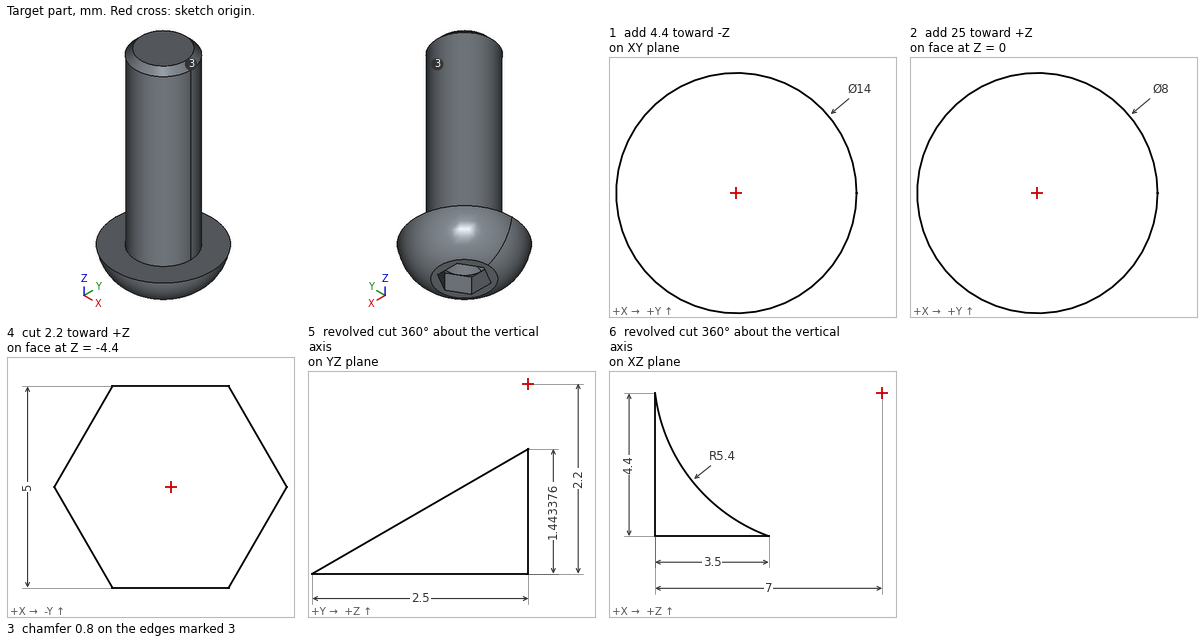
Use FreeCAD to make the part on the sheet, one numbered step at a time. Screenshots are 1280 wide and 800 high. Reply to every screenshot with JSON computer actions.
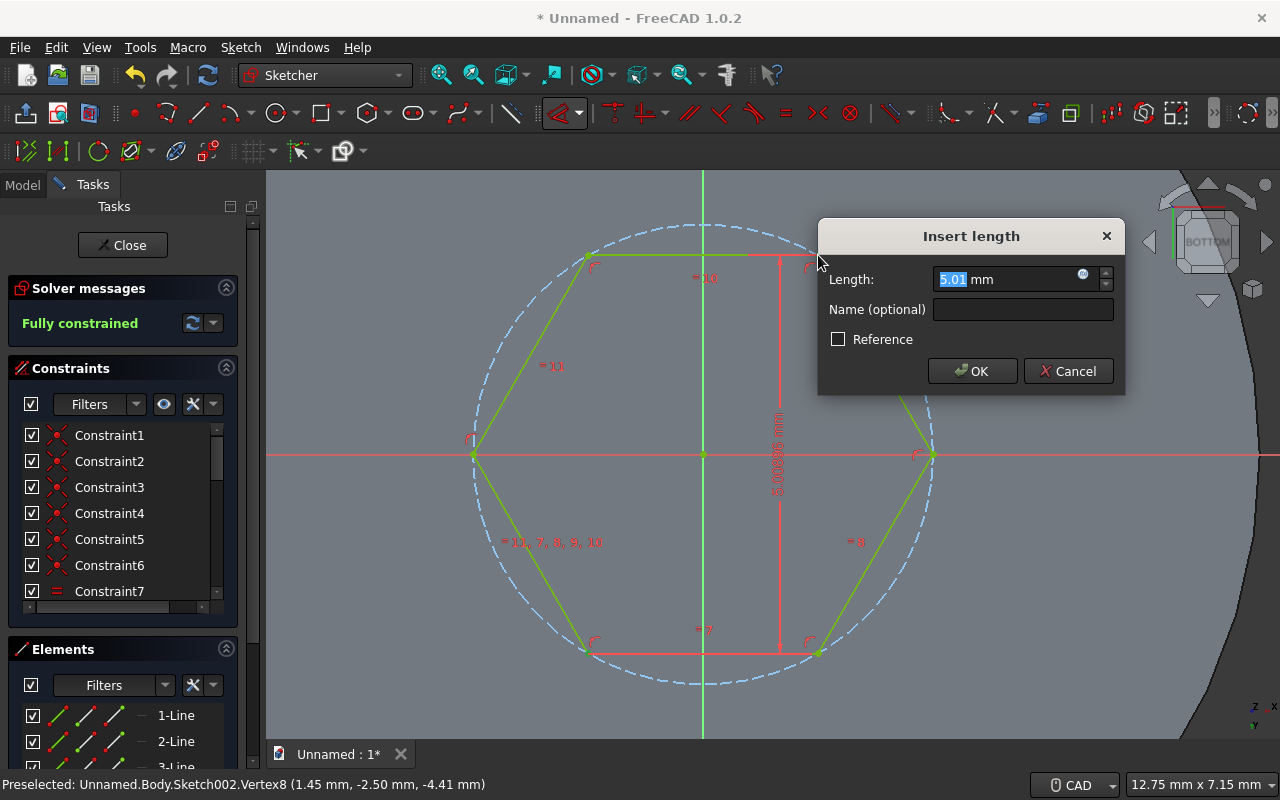
{"action": "type", "text": "5"}
{"action": "key", "text": "Return"}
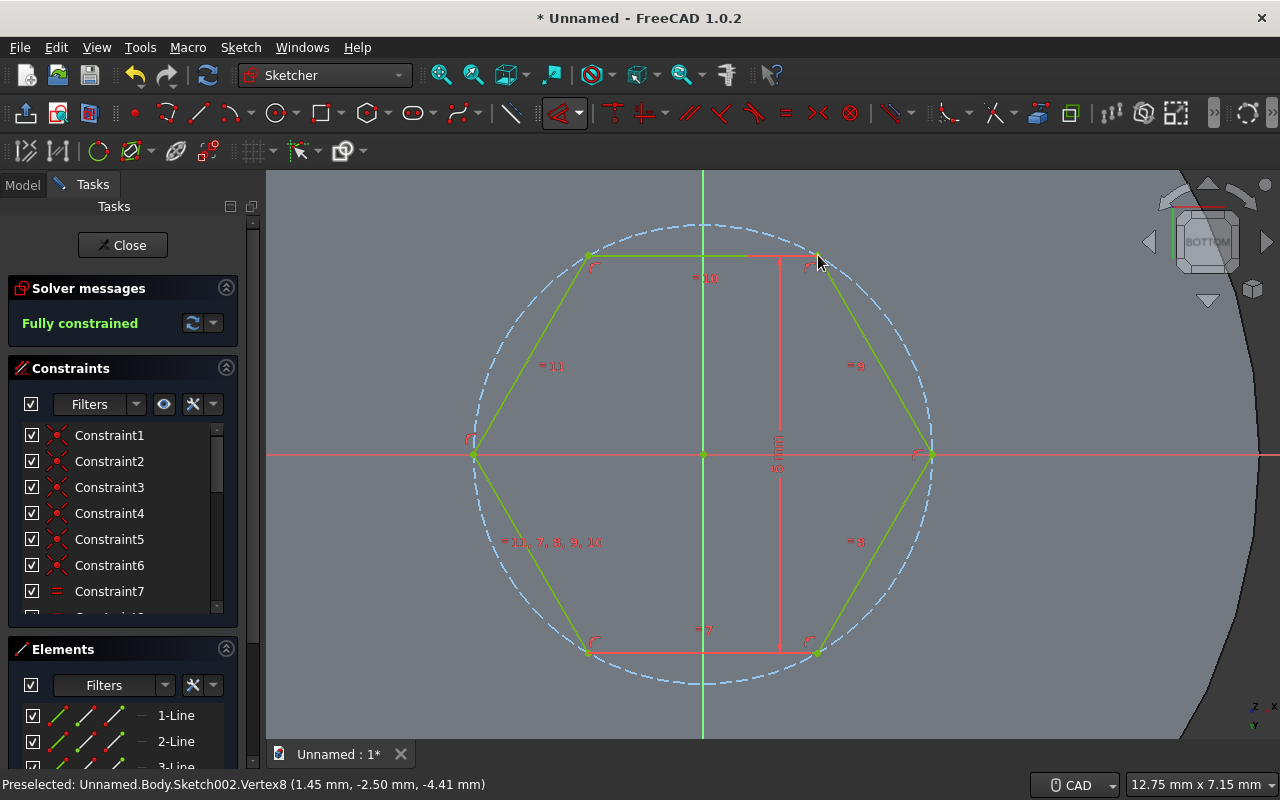
{"action": "left_click", "coordinate": [123, 245]}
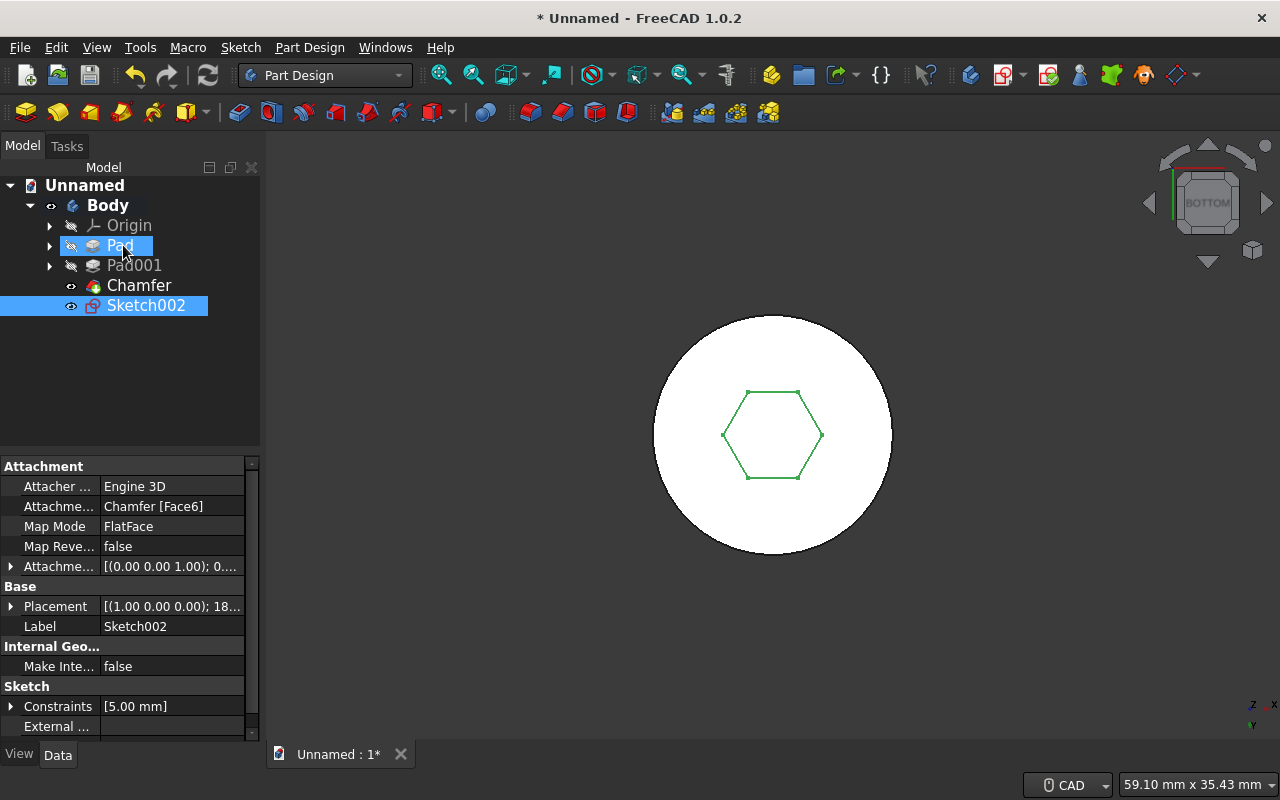
{"action": "left_click", "coordinate": [240, 112]}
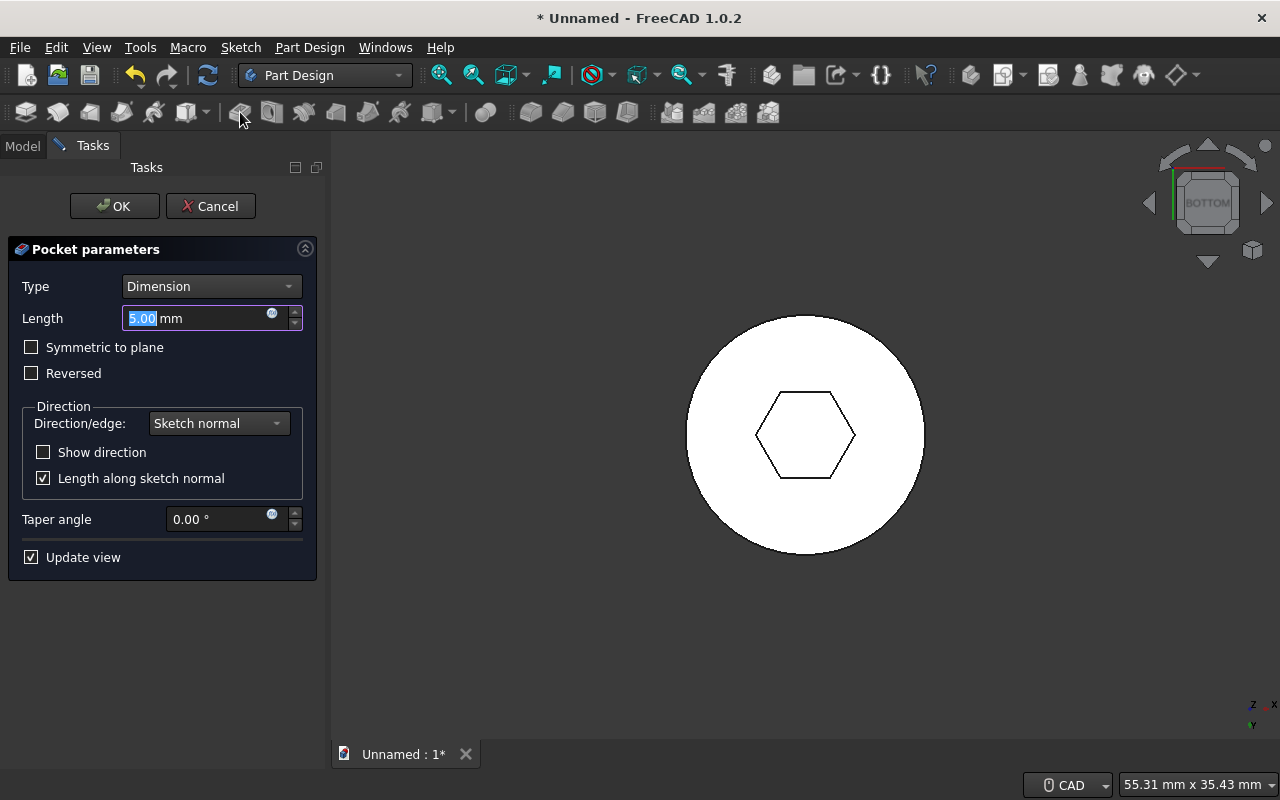
{"action": "type", "text": "2.2"}
{"action": "key", "text": "Tab"}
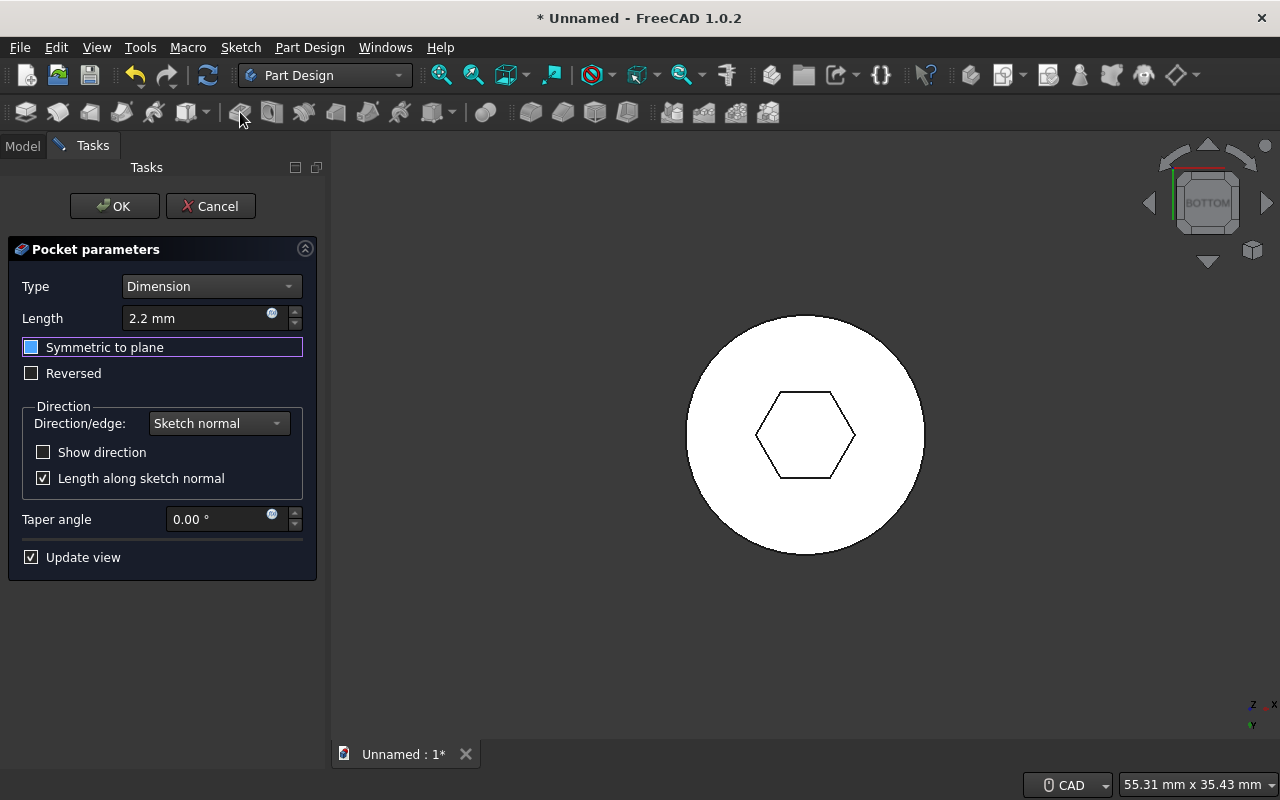
{"action": "left_click", "coordinate": [115, 206]}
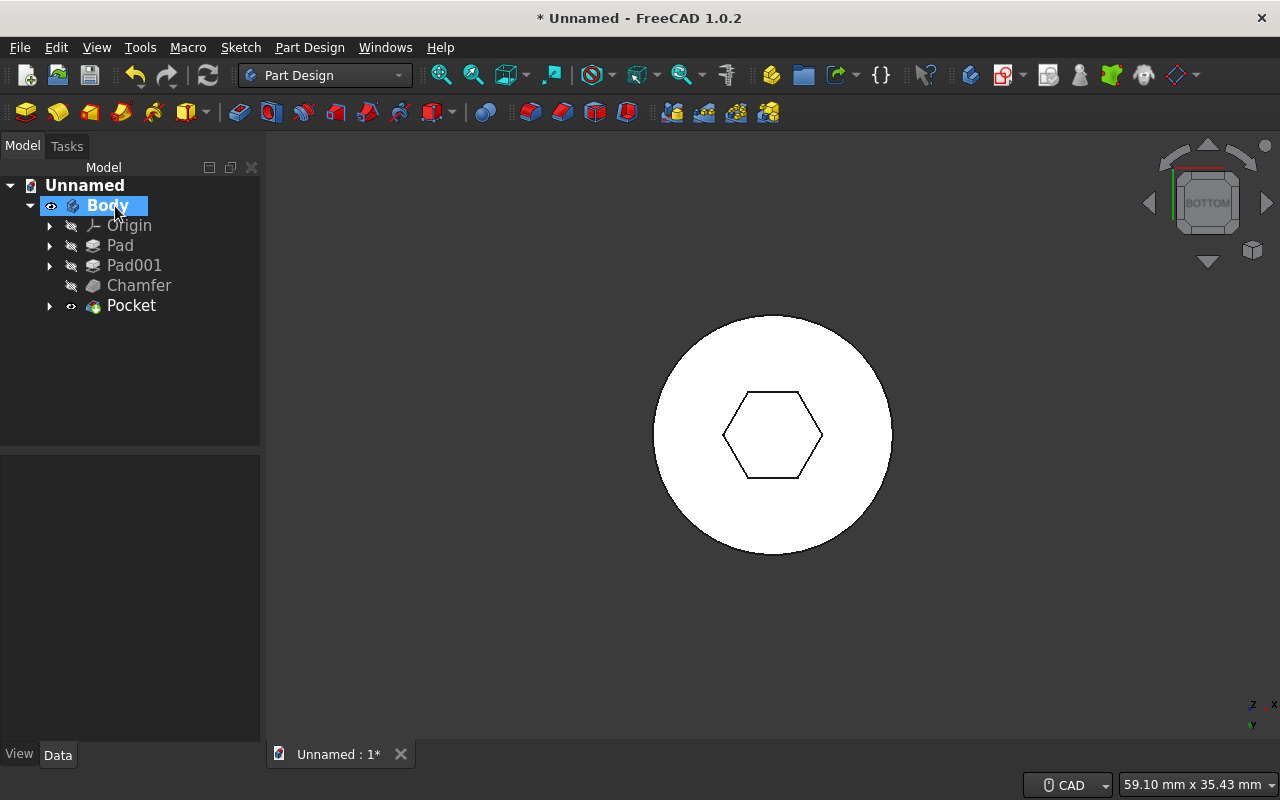
{"action": "left_click", "coordinate": [442, 76]}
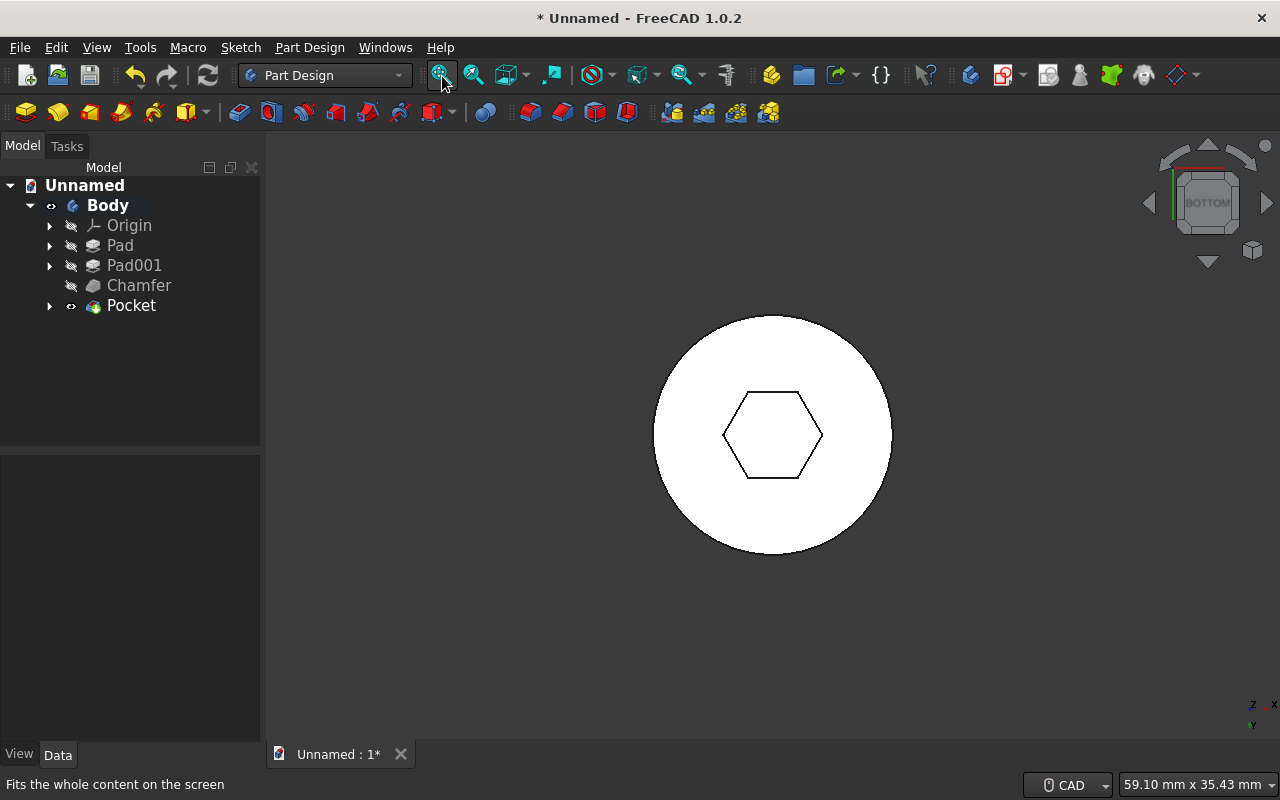
{"action": "left_click", "coordinate": [1004, 76]}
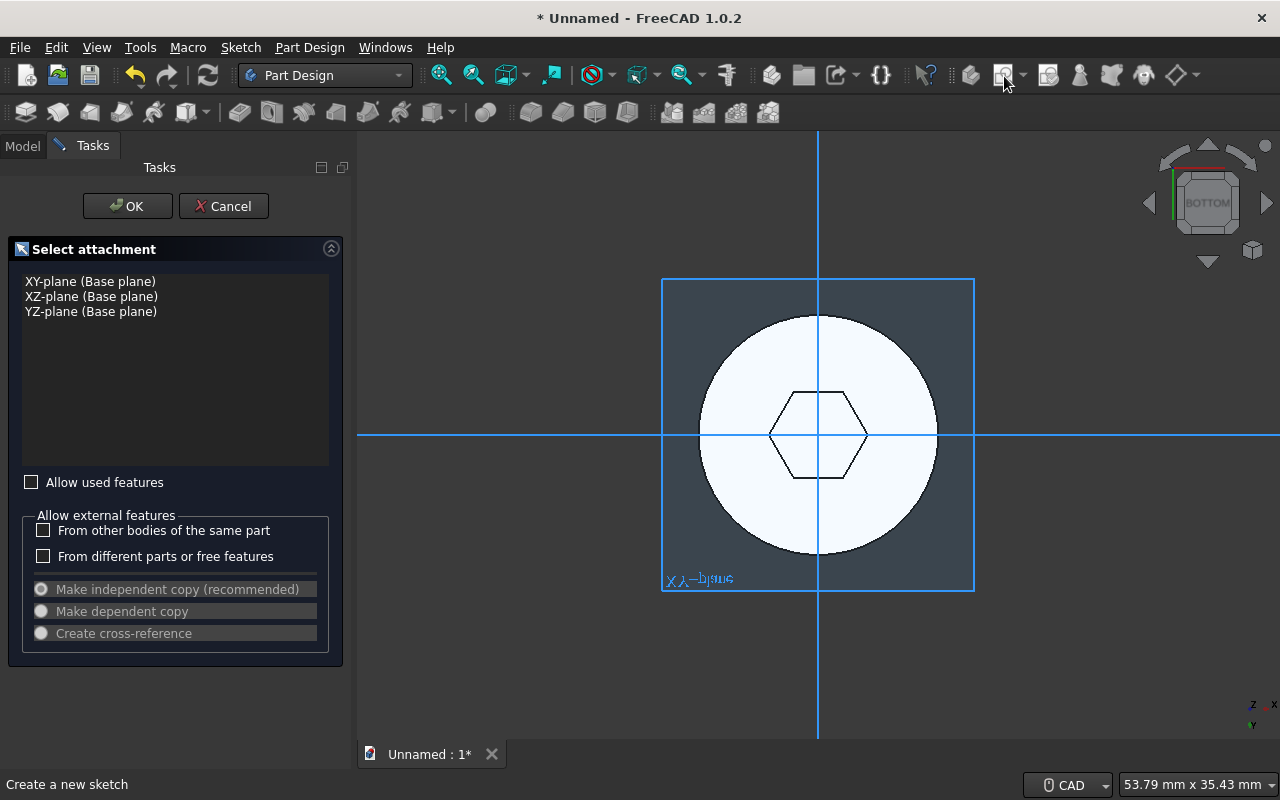
{"action": "left_click", "coordinate": [82, 312]}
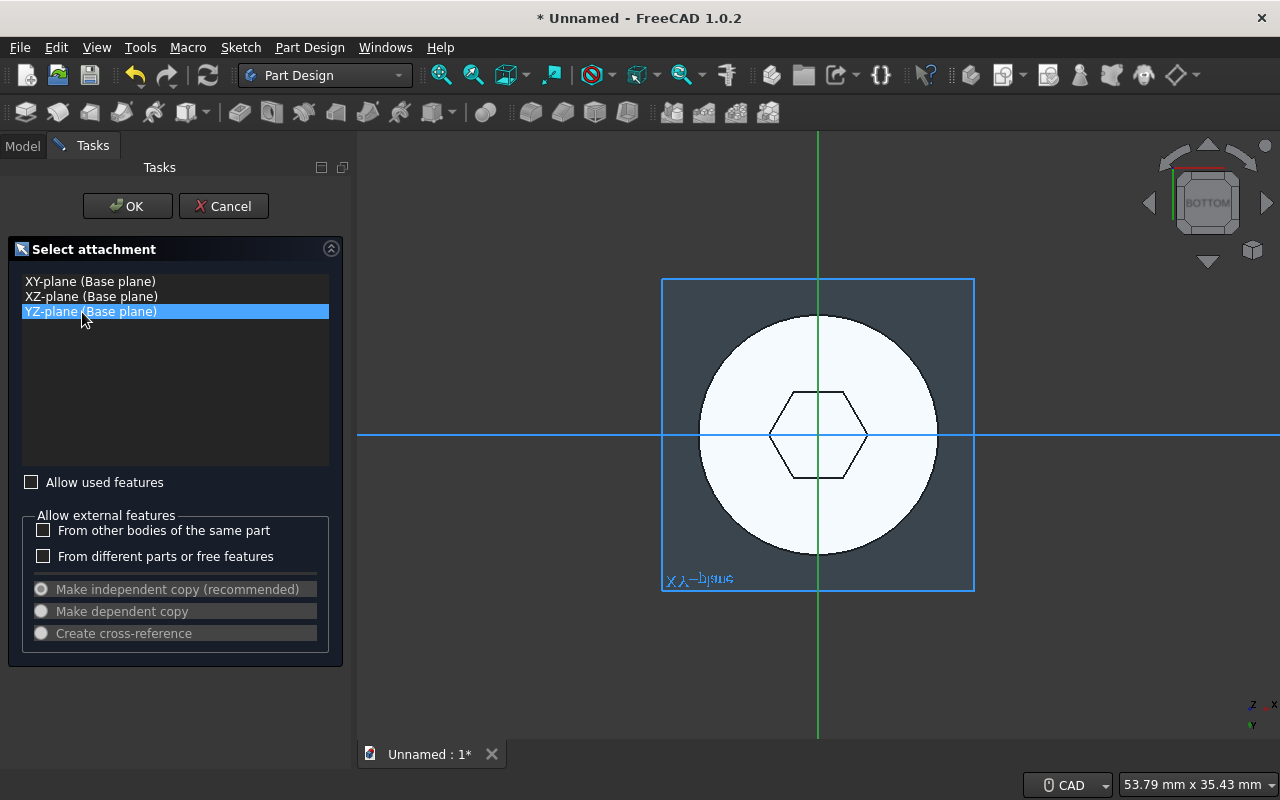
{"action": "left_click", "coordinate": [128, 206]}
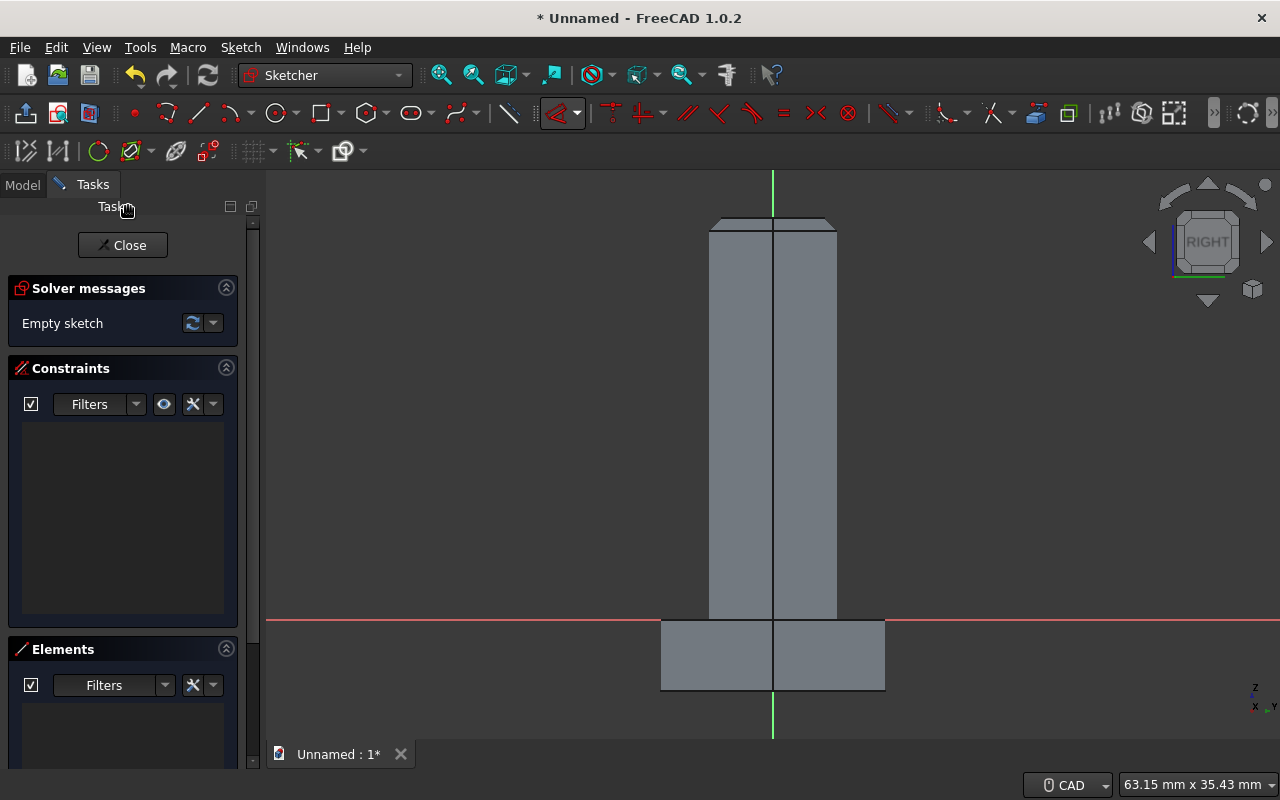
{"action": "left_click", "coordinate": [90, 114]}